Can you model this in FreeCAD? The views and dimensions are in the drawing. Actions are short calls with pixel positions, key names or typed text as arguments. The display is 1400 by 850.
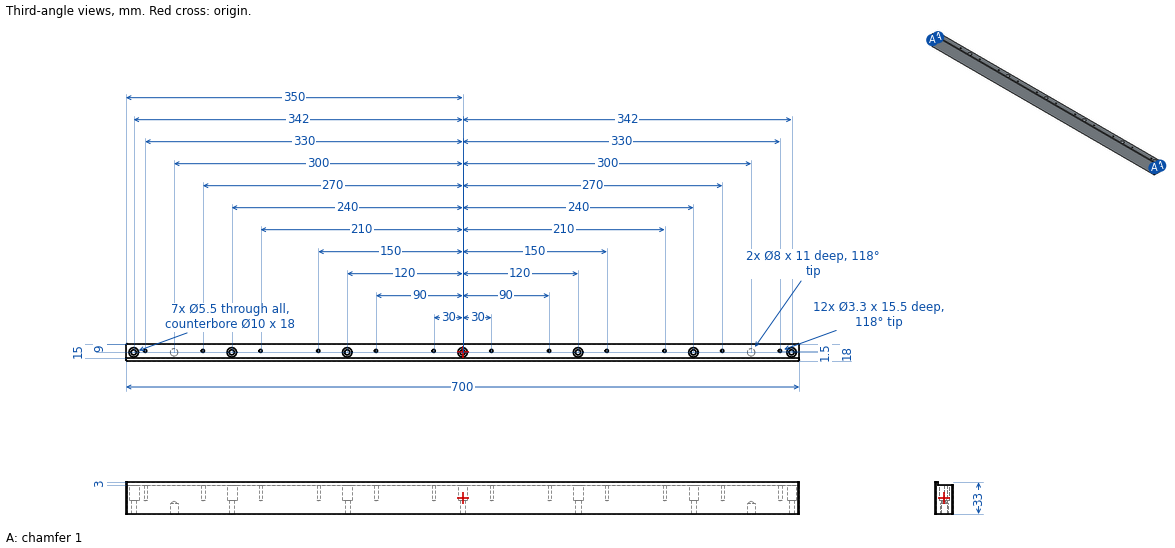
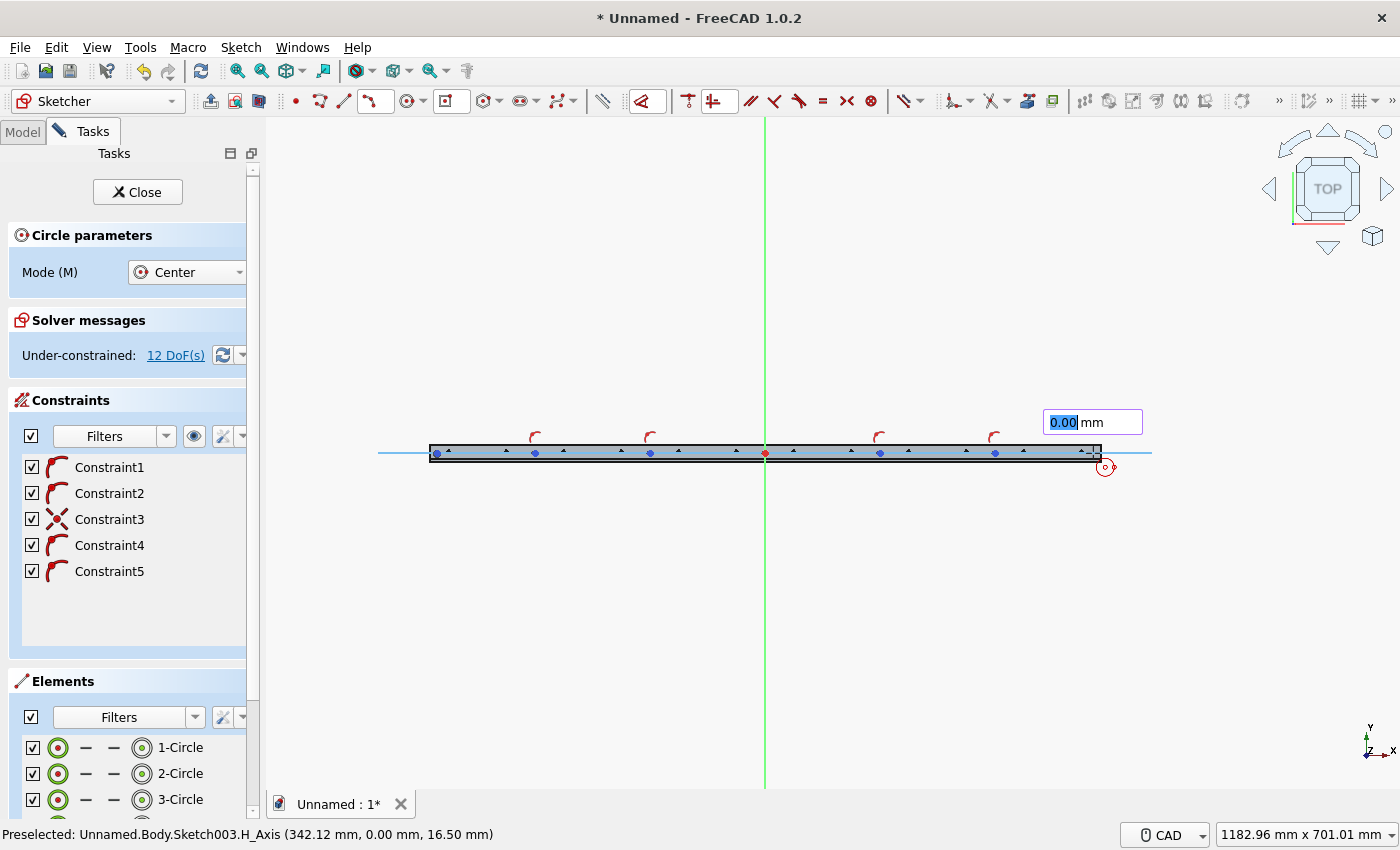
scroll(1094, 451, up, 10)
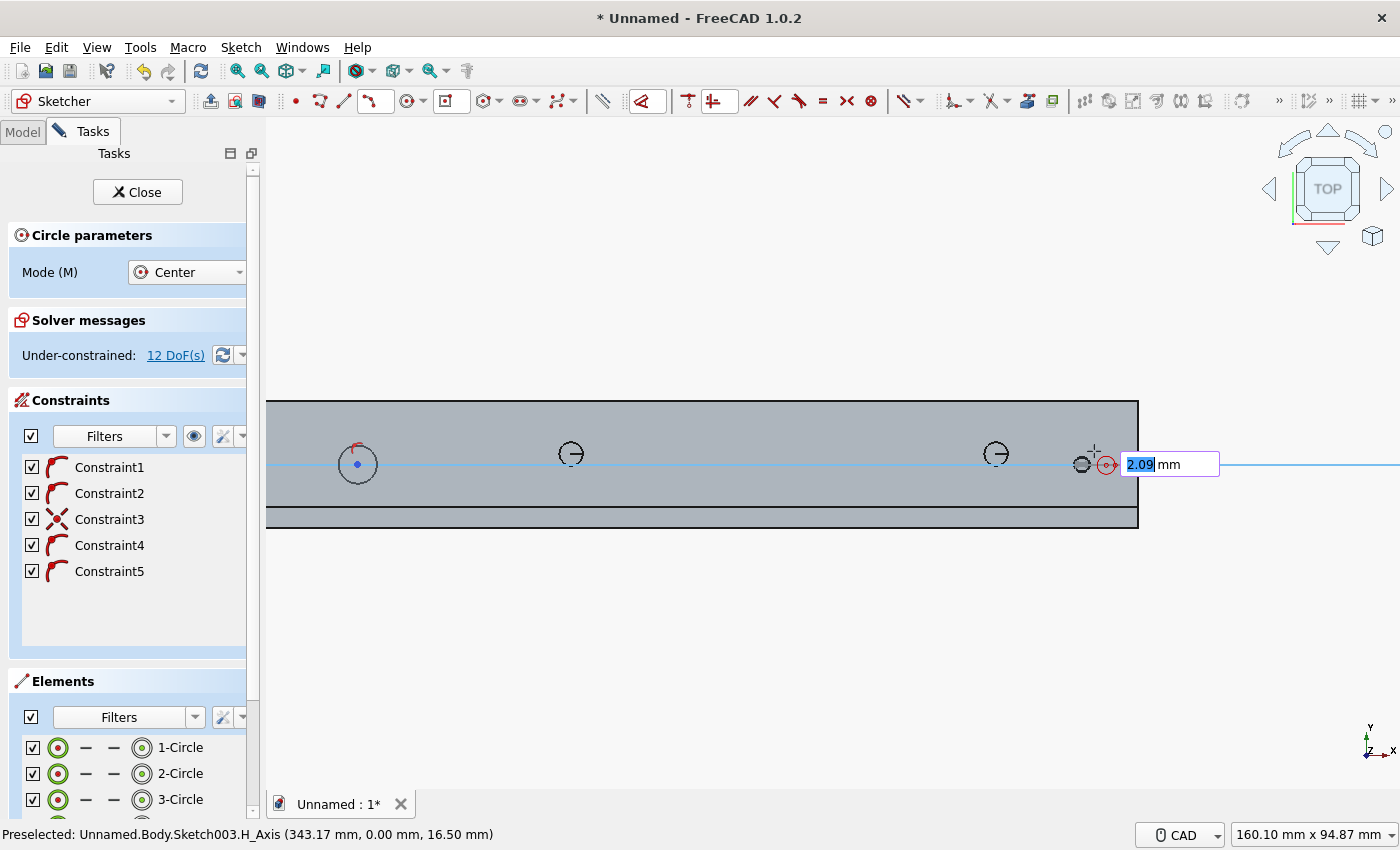
click(1088, 446)
key(Escape)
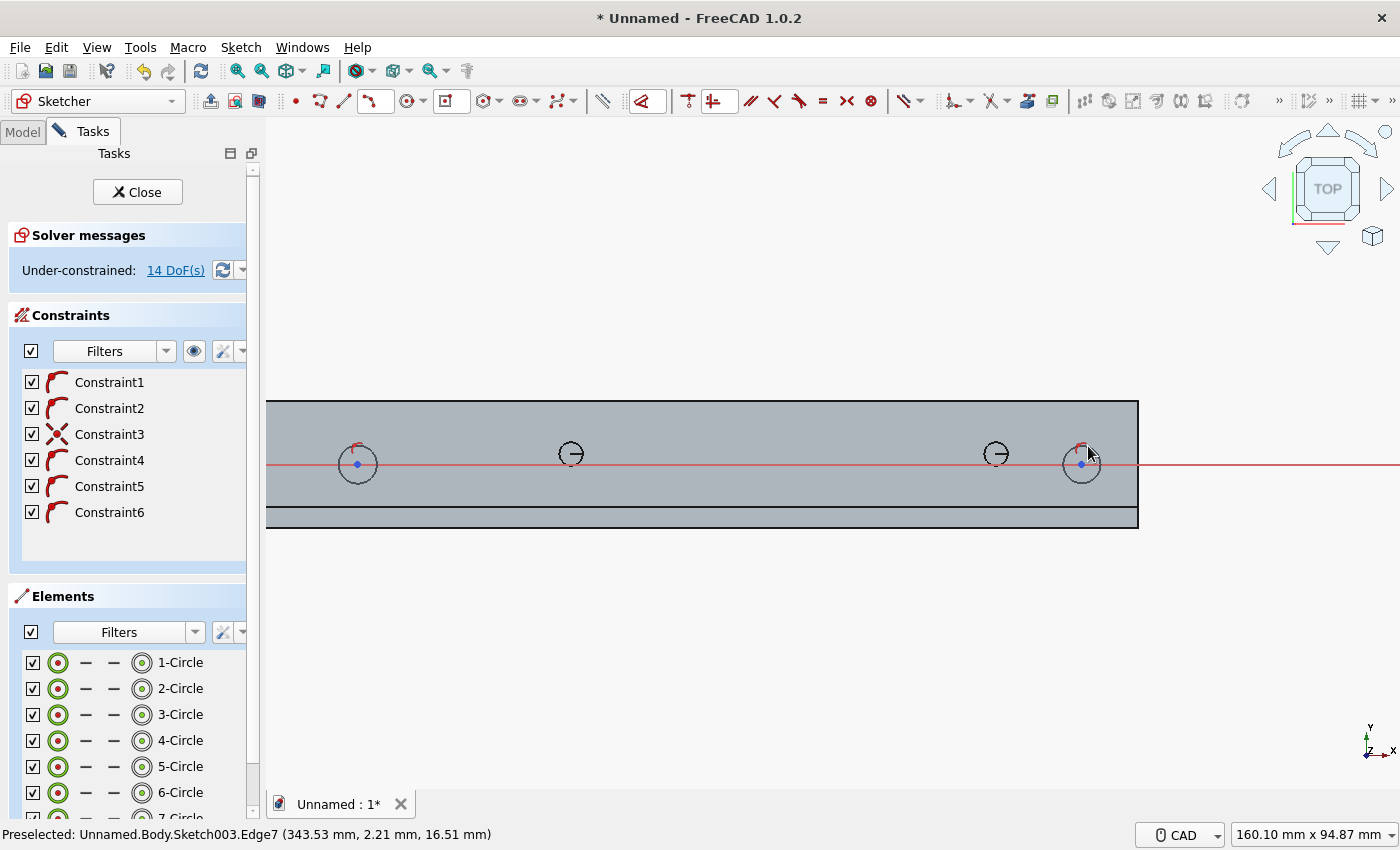
scroll(1094, 451, down, 10)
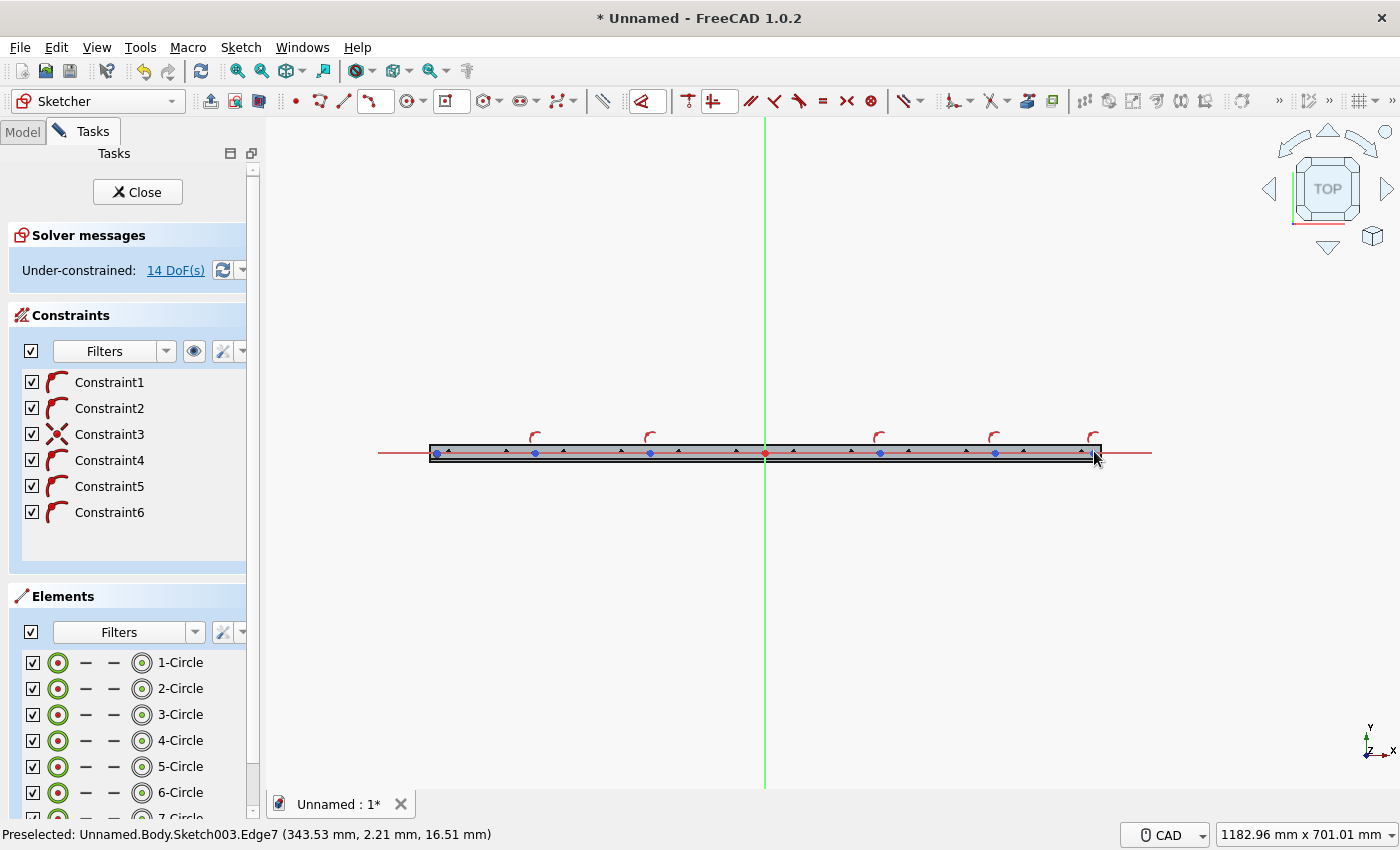
scroll(439, 452, up, 11)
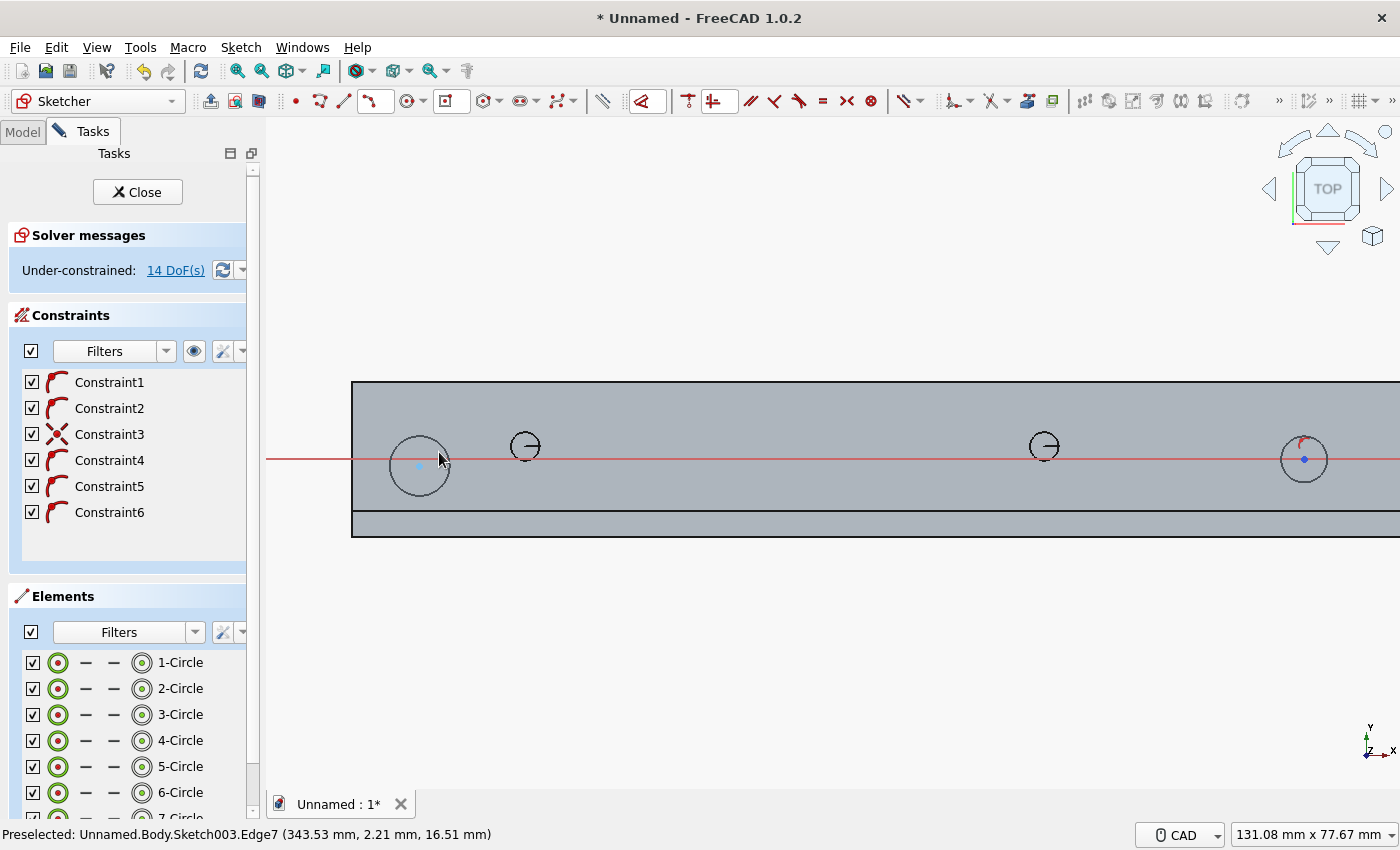
click(441, 445)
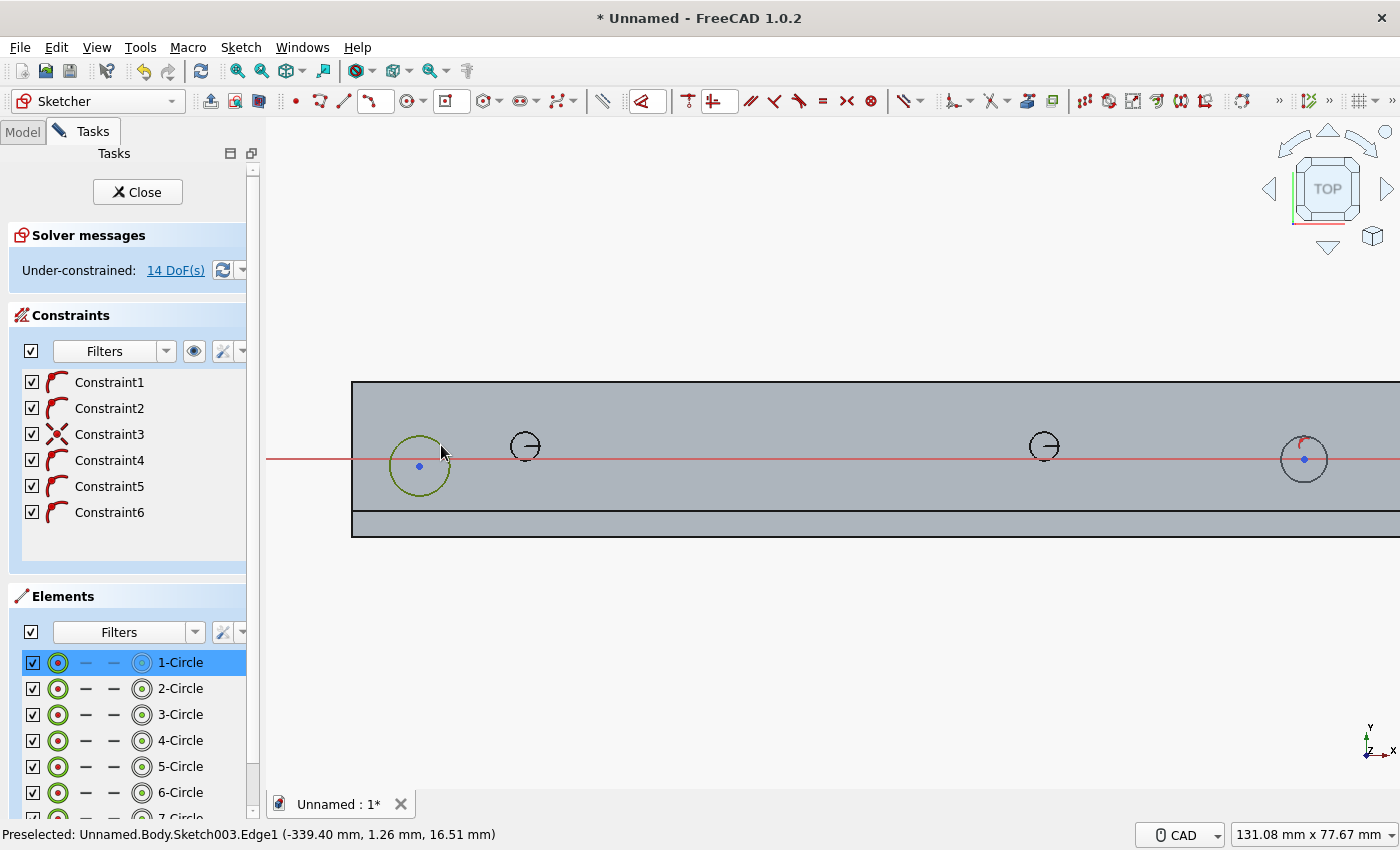
scroll(439, 452, down, 11)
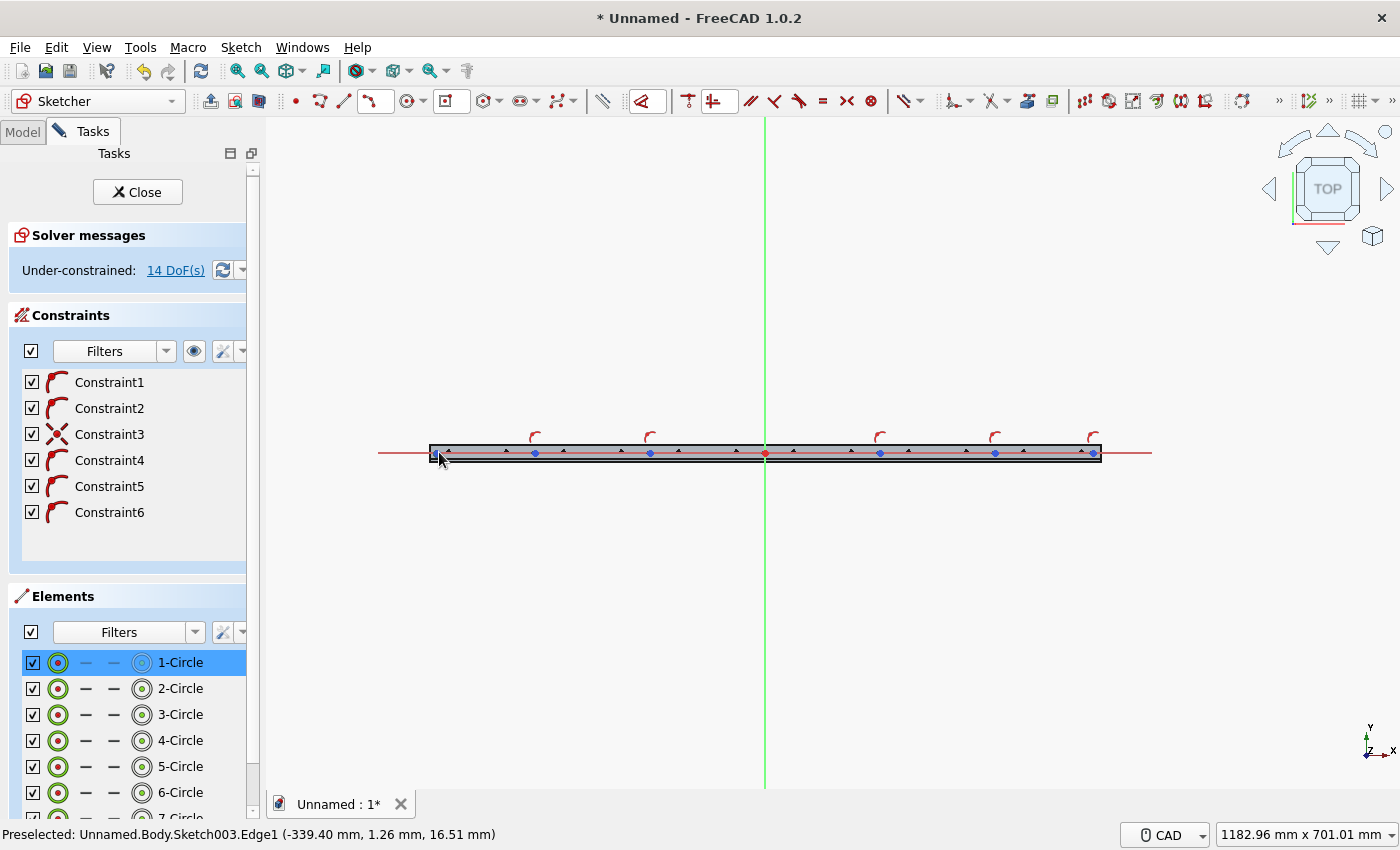
scroll(537, 451, up, 11)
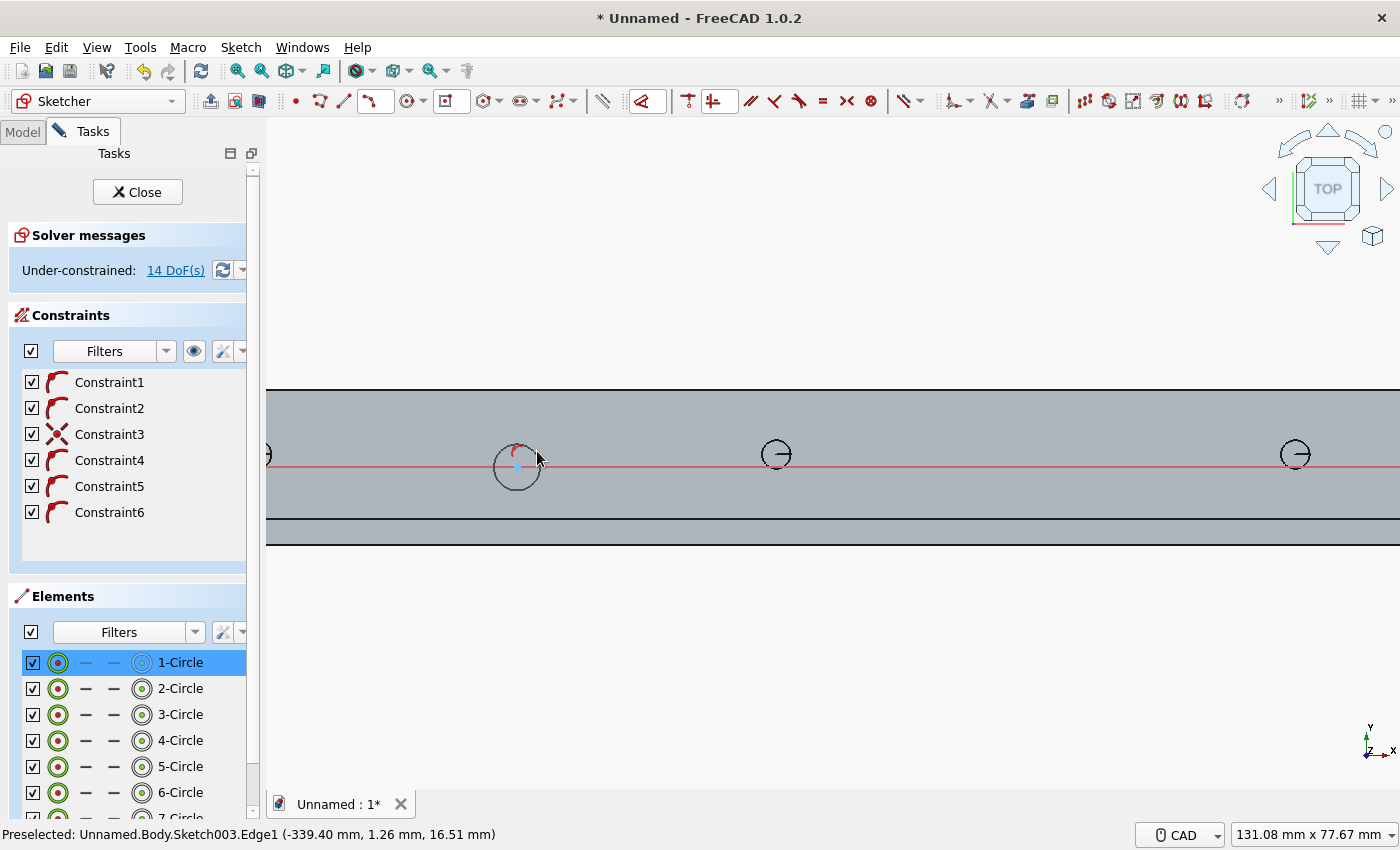
click(533, 451)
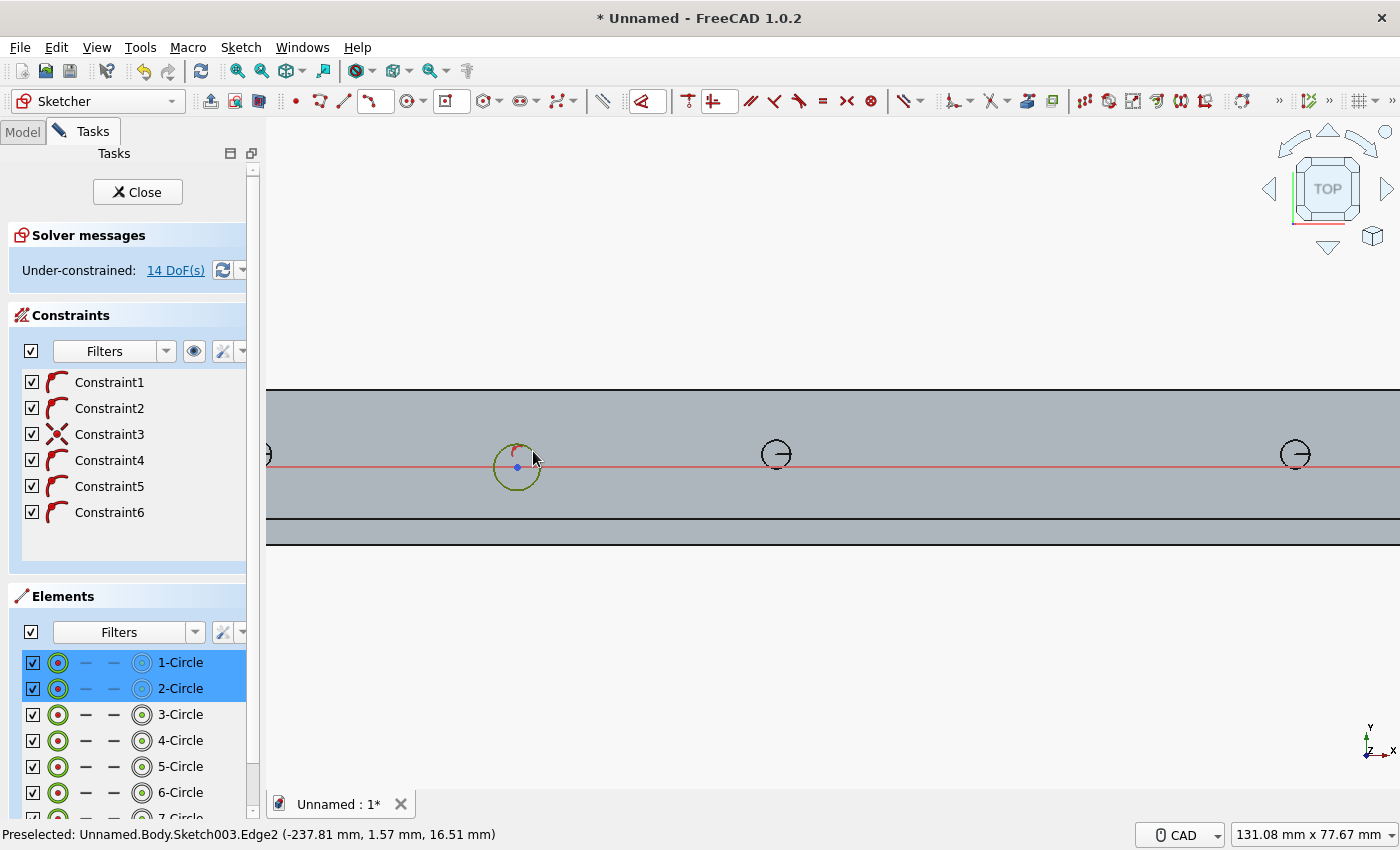
scroll(537, 451, down, 11)